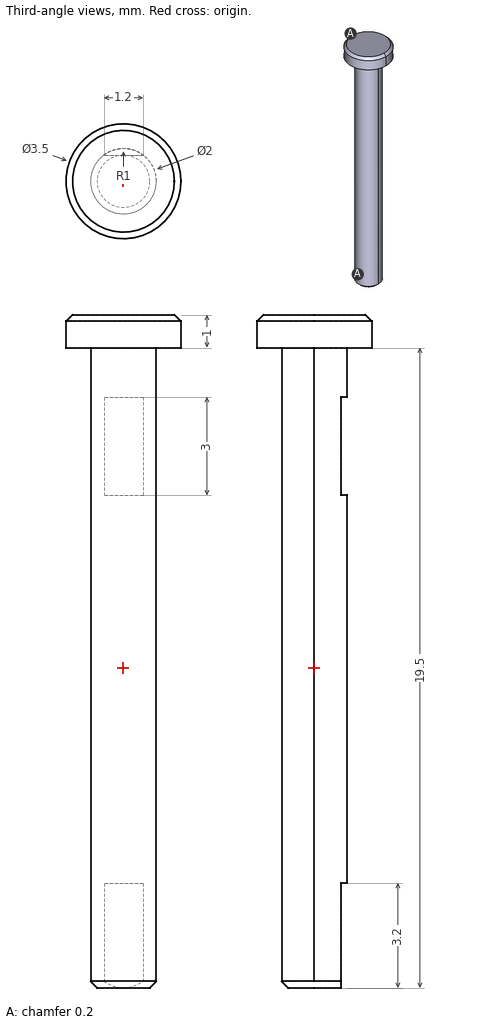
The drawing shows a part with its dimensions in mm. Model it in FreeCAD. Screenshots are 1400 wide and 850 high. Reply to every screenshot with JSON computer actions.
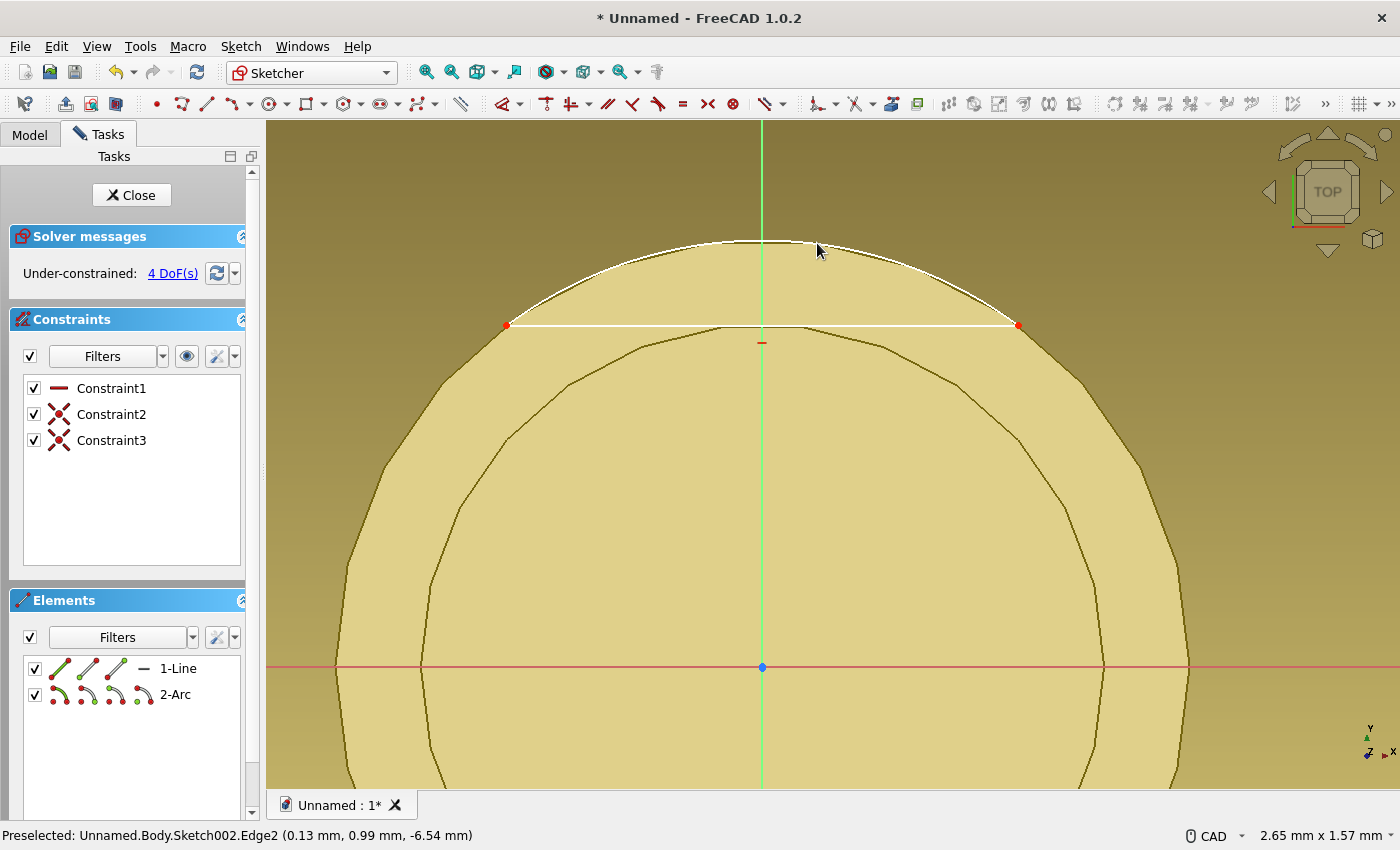
{"action": "left_click_drag", "start_coordinate": [752, 657], "coordinate": [773, 678]}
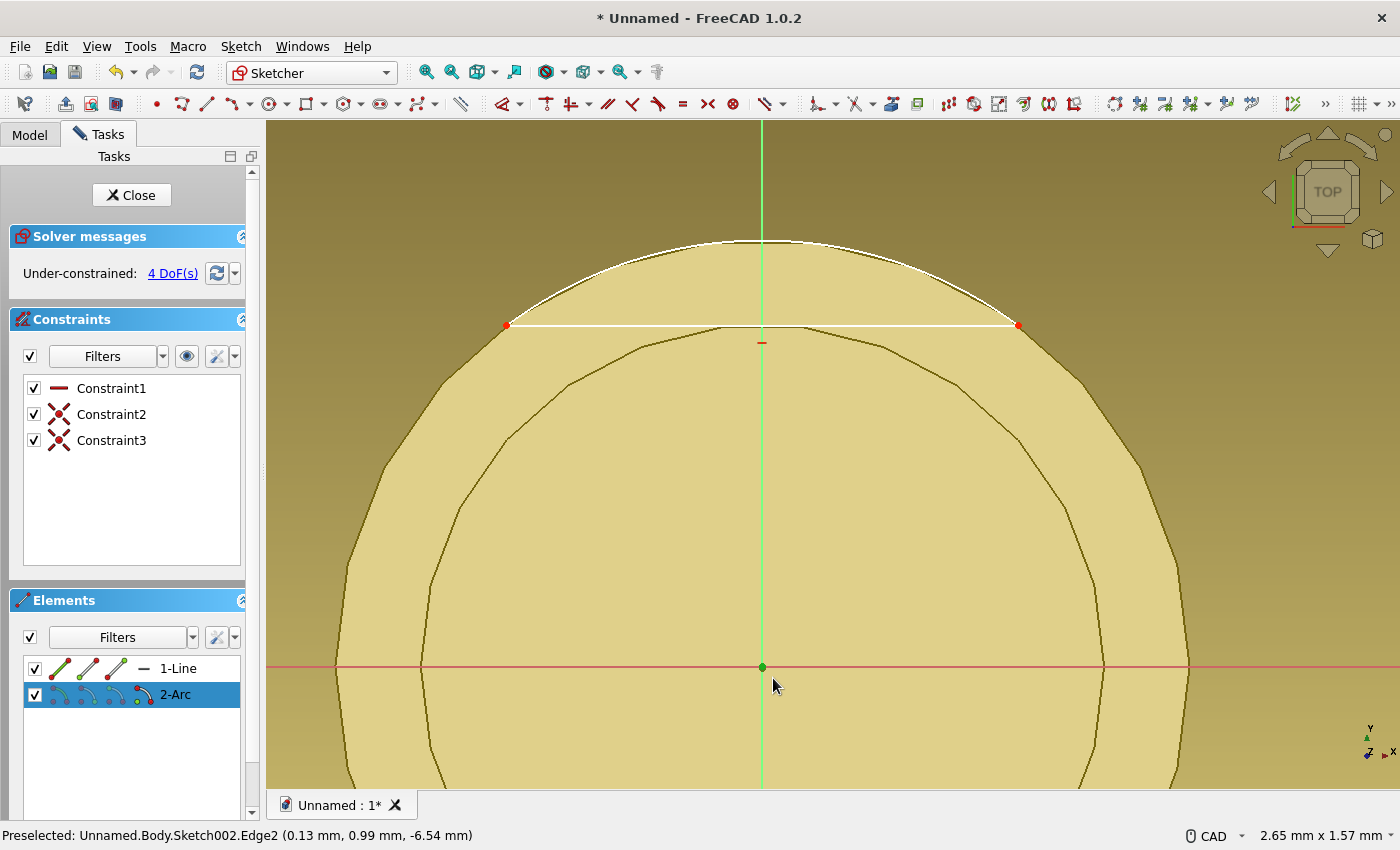
{"action": "key", "text": "c"}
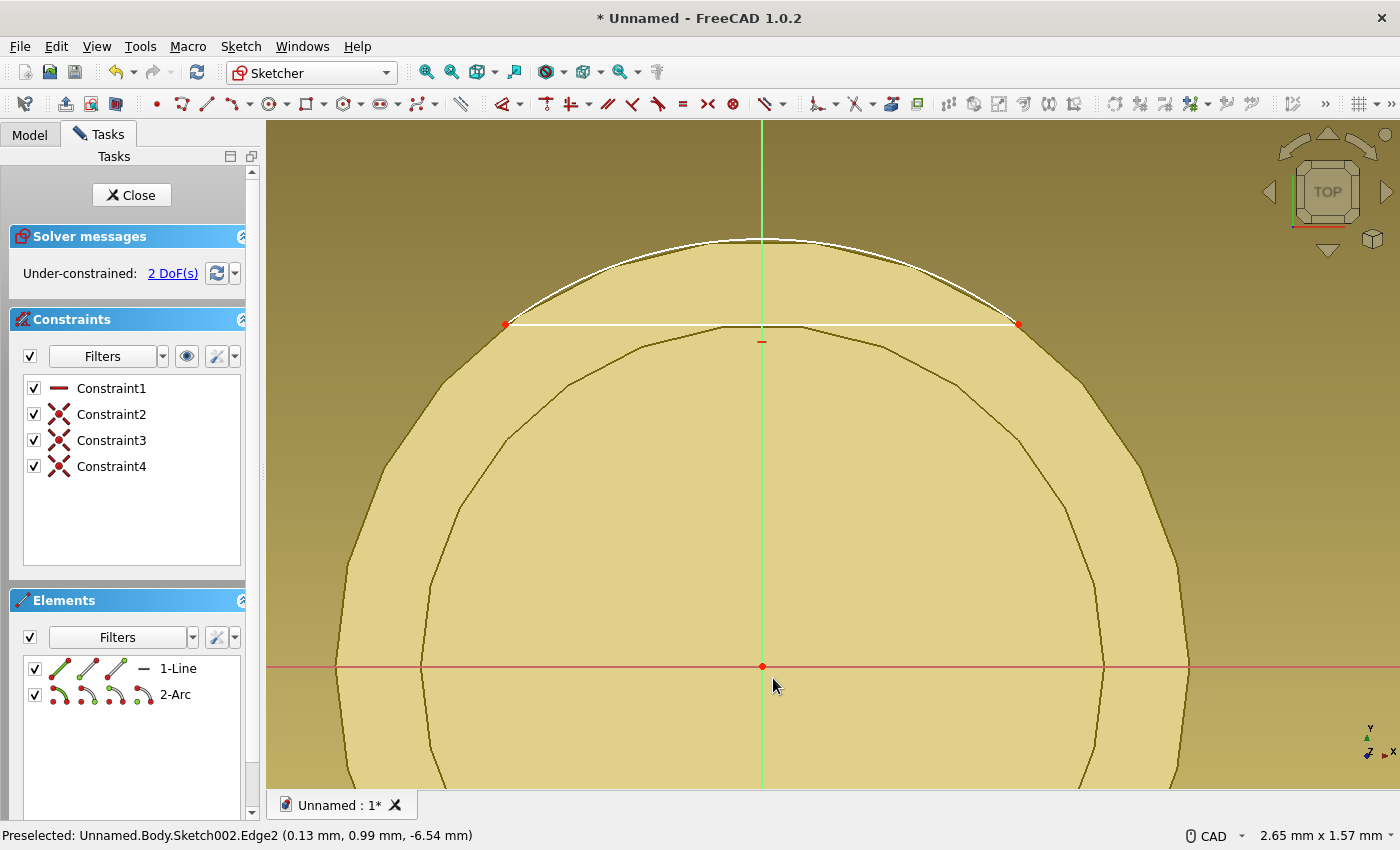
{"action": "left_click", "coordinate": [871, 253]}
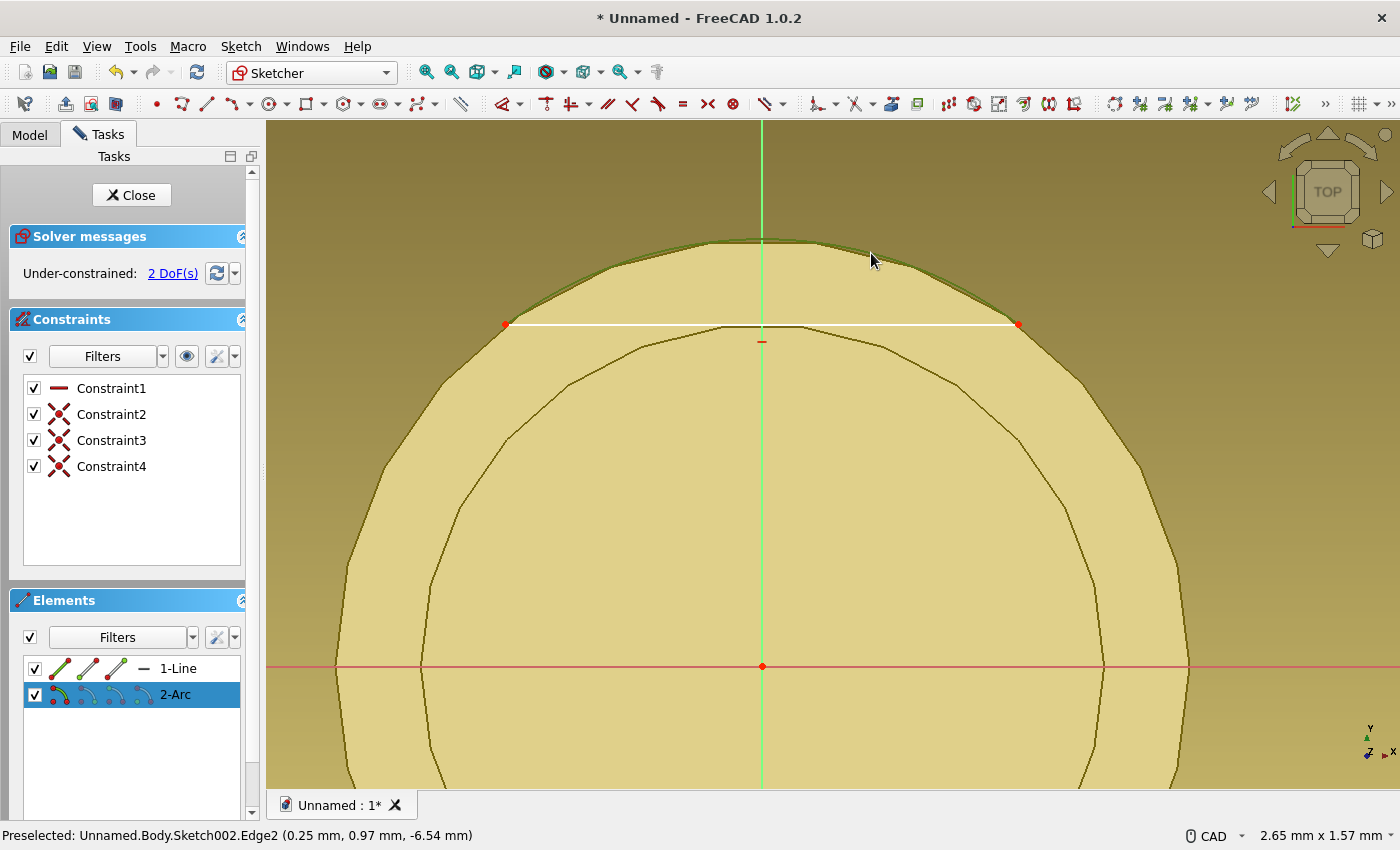
{"action": "key", "text": "k r"}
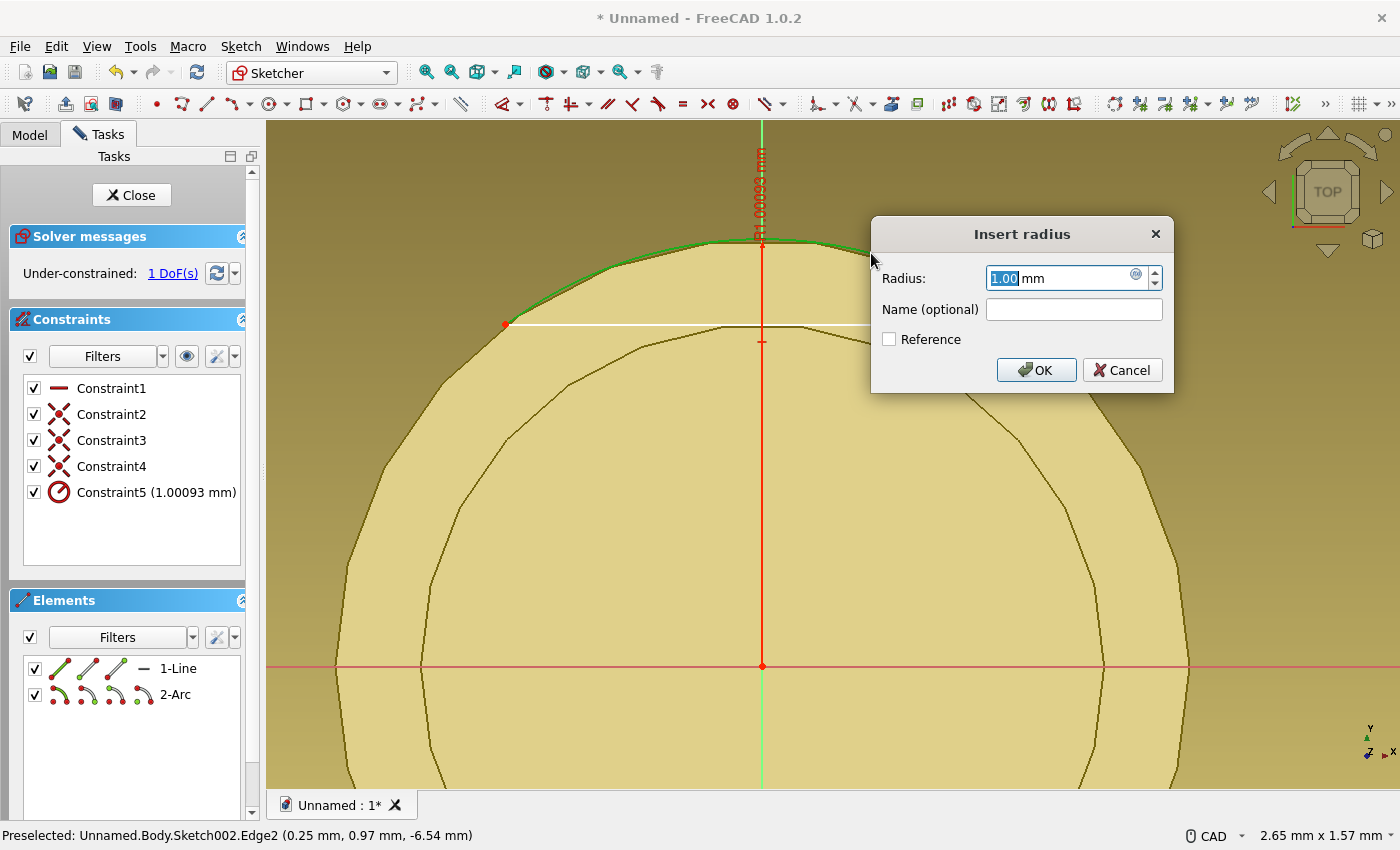
{"action": "type", "text": "1"}
{"action": "key", "text": "Return"}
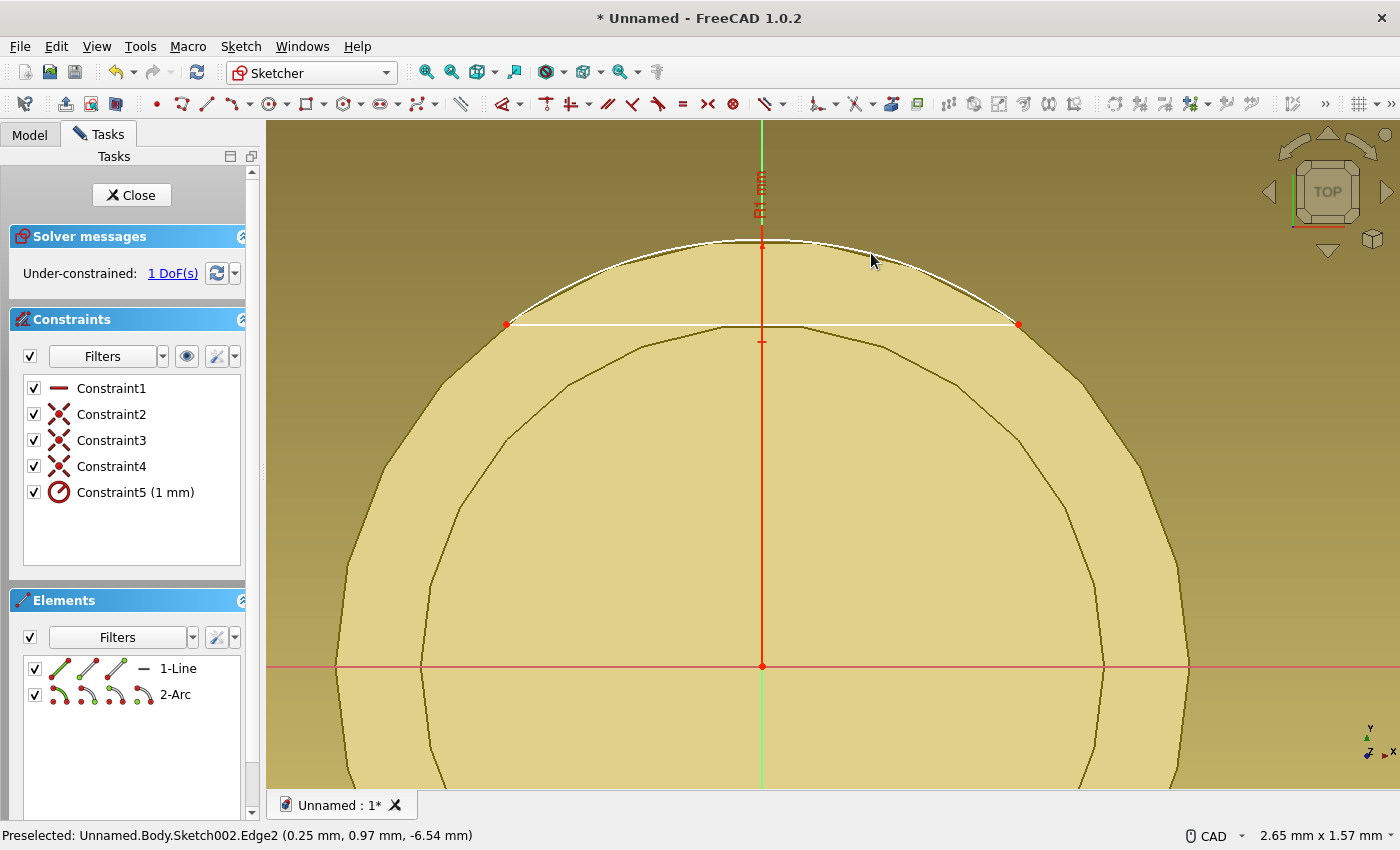
{"action": "left_click", "coordinate": [865, 325]}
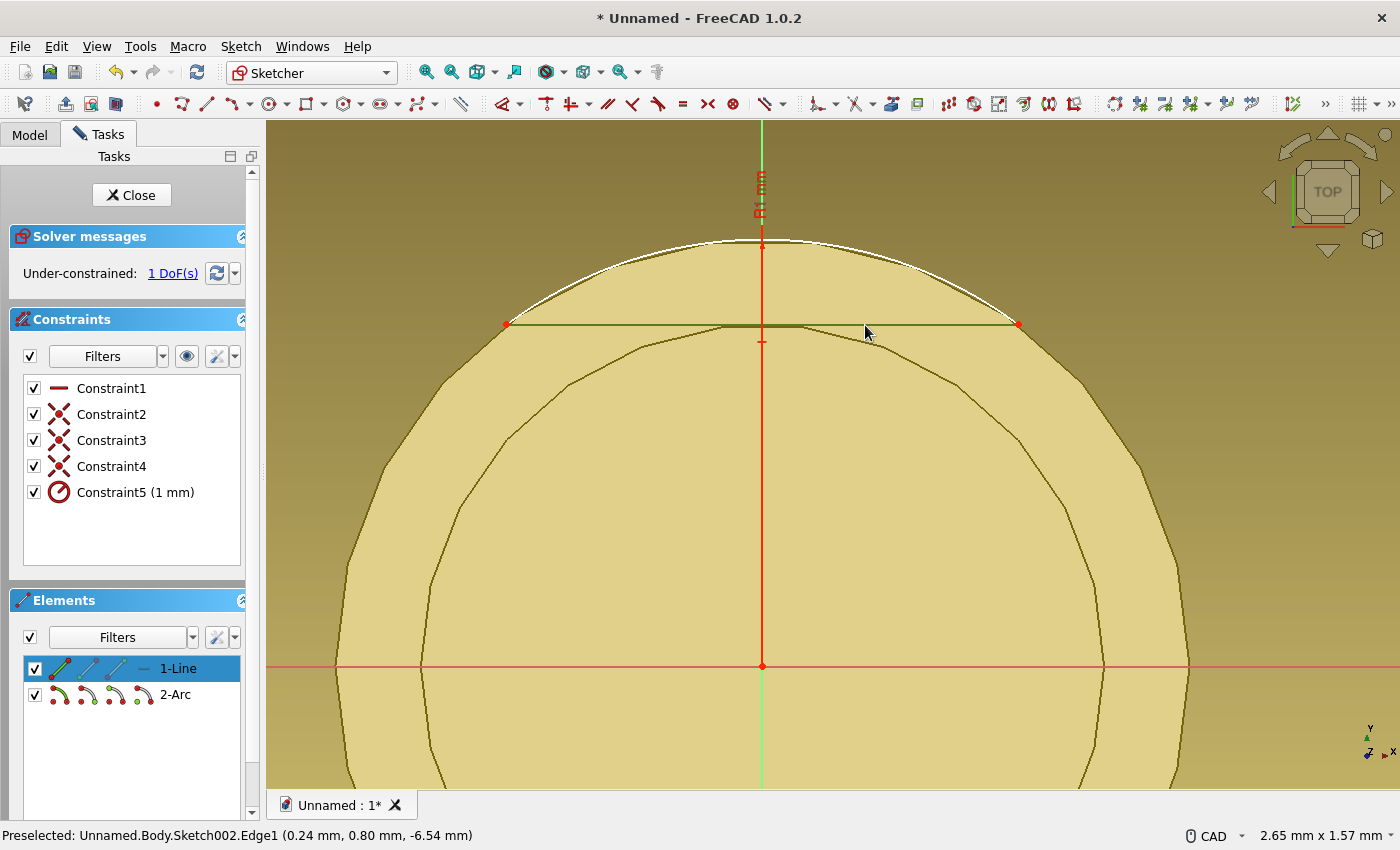
{"action": "key", "text": "l"}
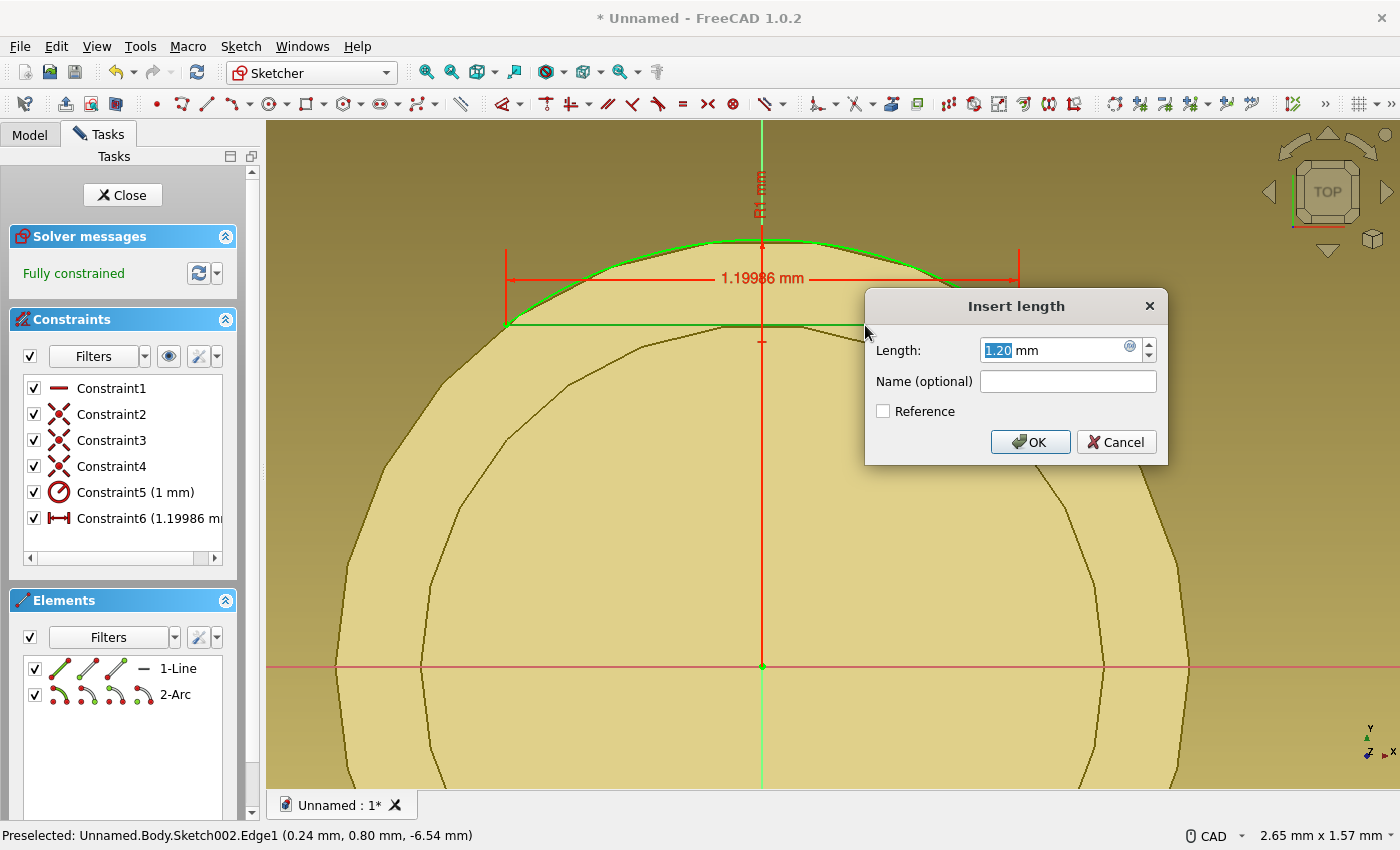
{"action": "type", "text": "1.2"}
{"action": "key", "text": "Return"}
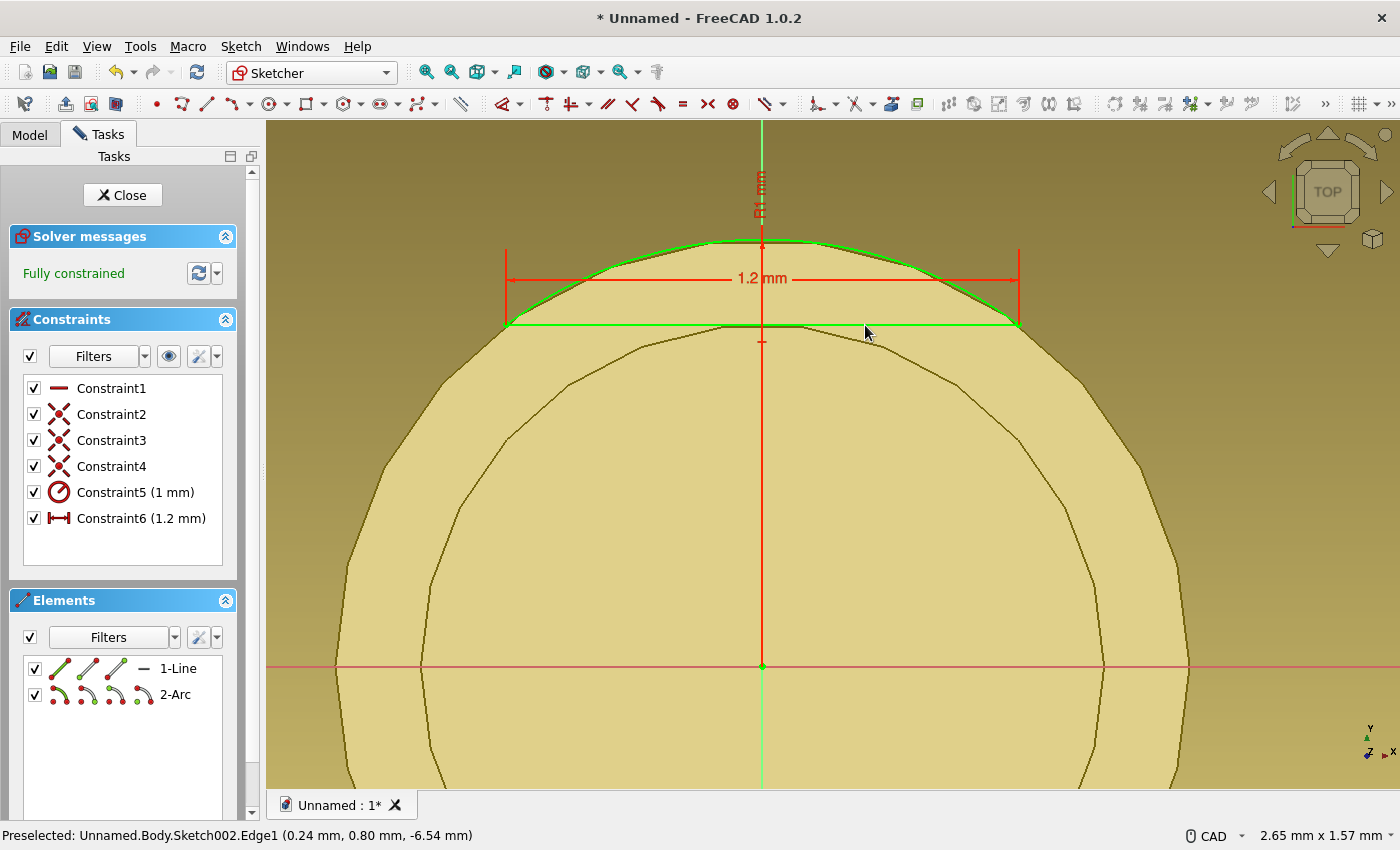
{"action": "left_click", "coordinate": [123, 195]}